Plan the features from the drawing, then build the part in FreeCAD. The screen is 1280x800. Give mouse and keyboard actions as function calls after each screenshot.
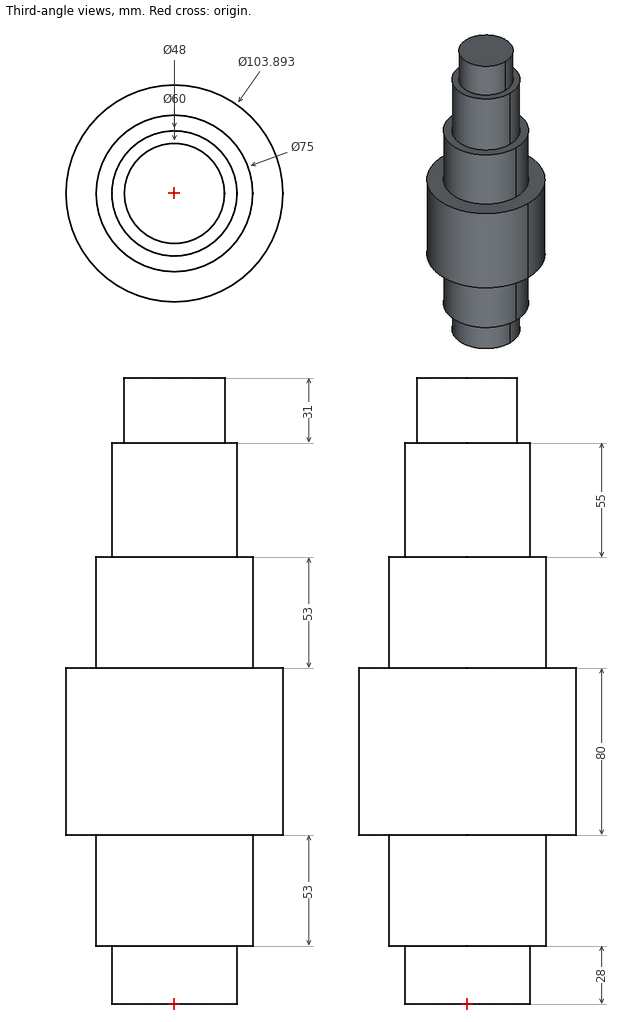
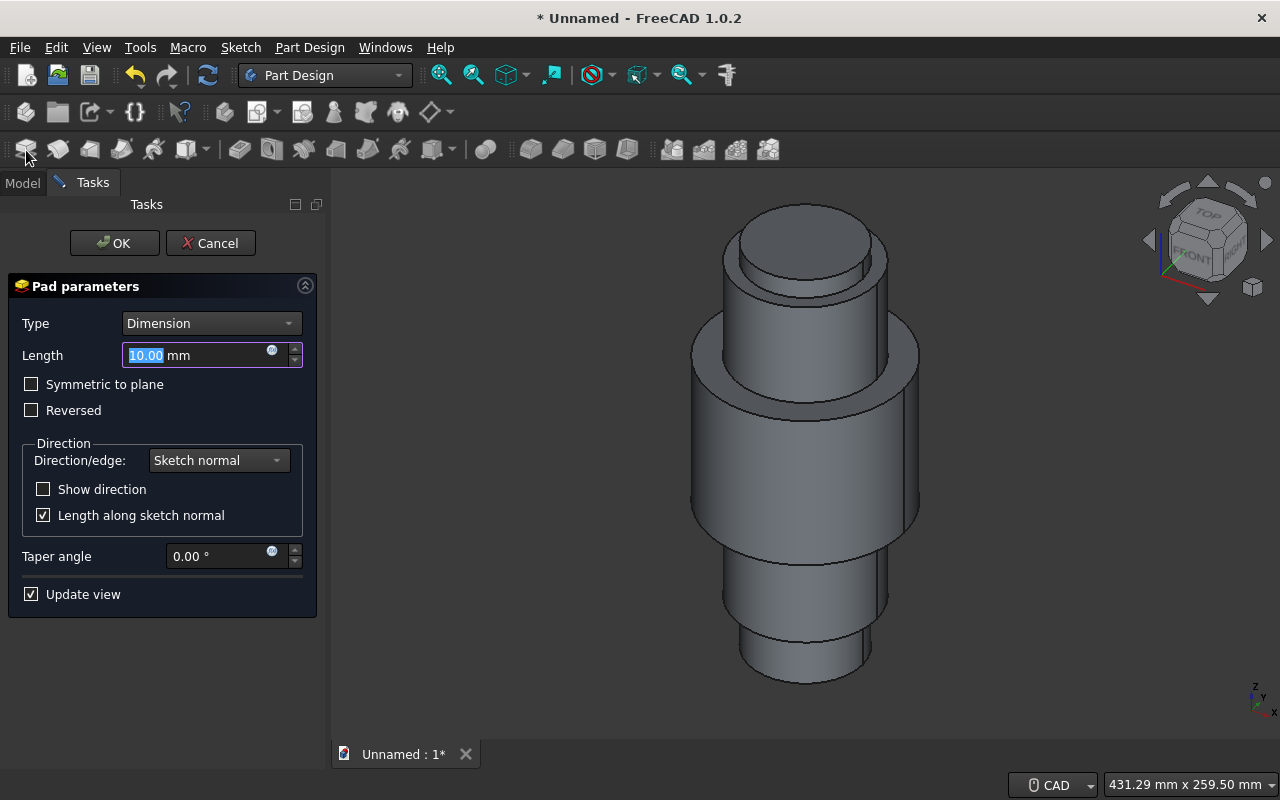
text(55)
key(Tab)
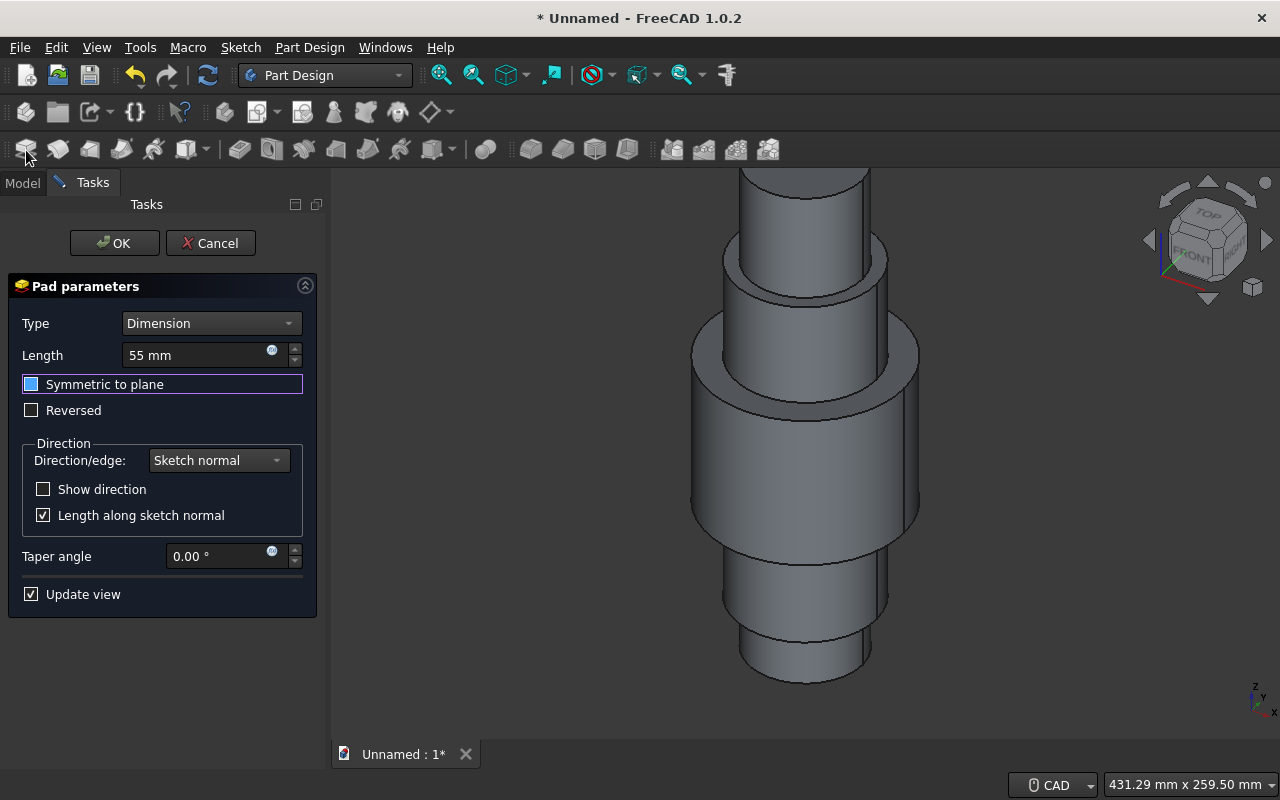
click(115, 243)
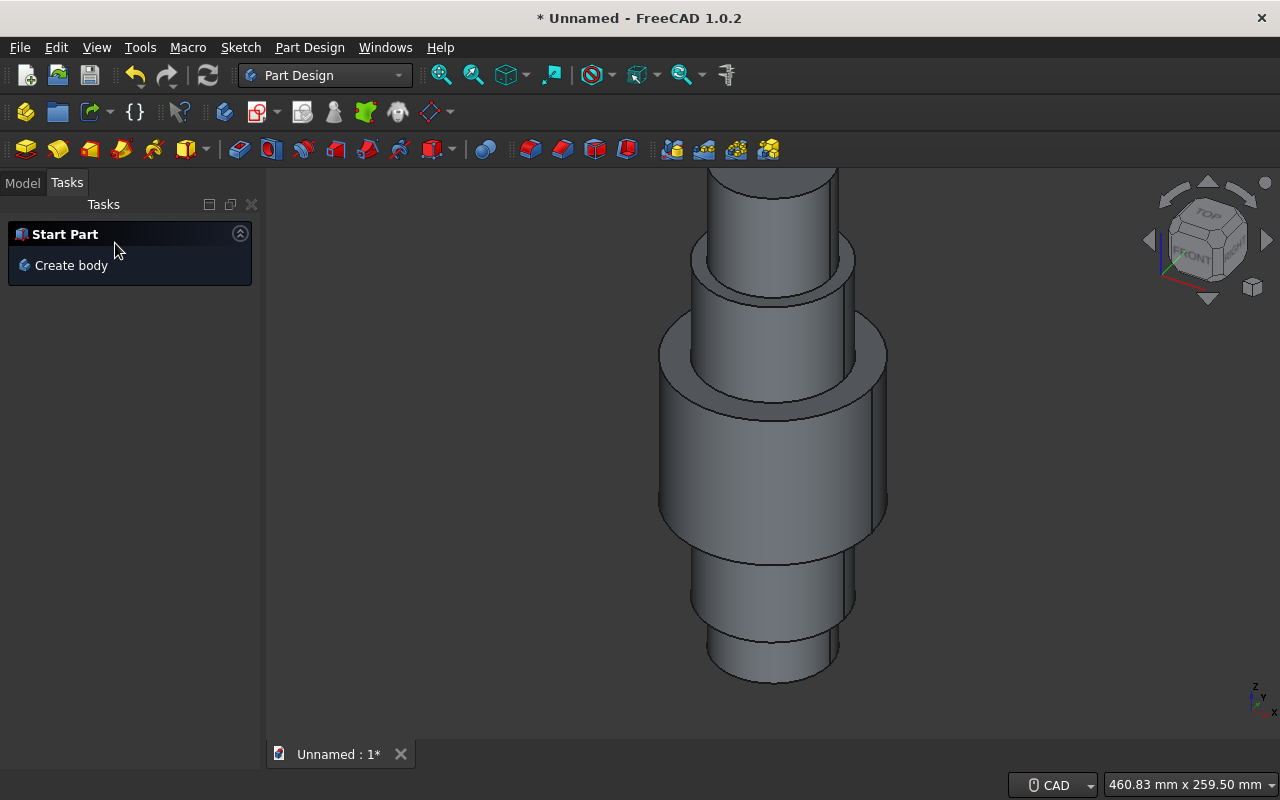
click(442, 76)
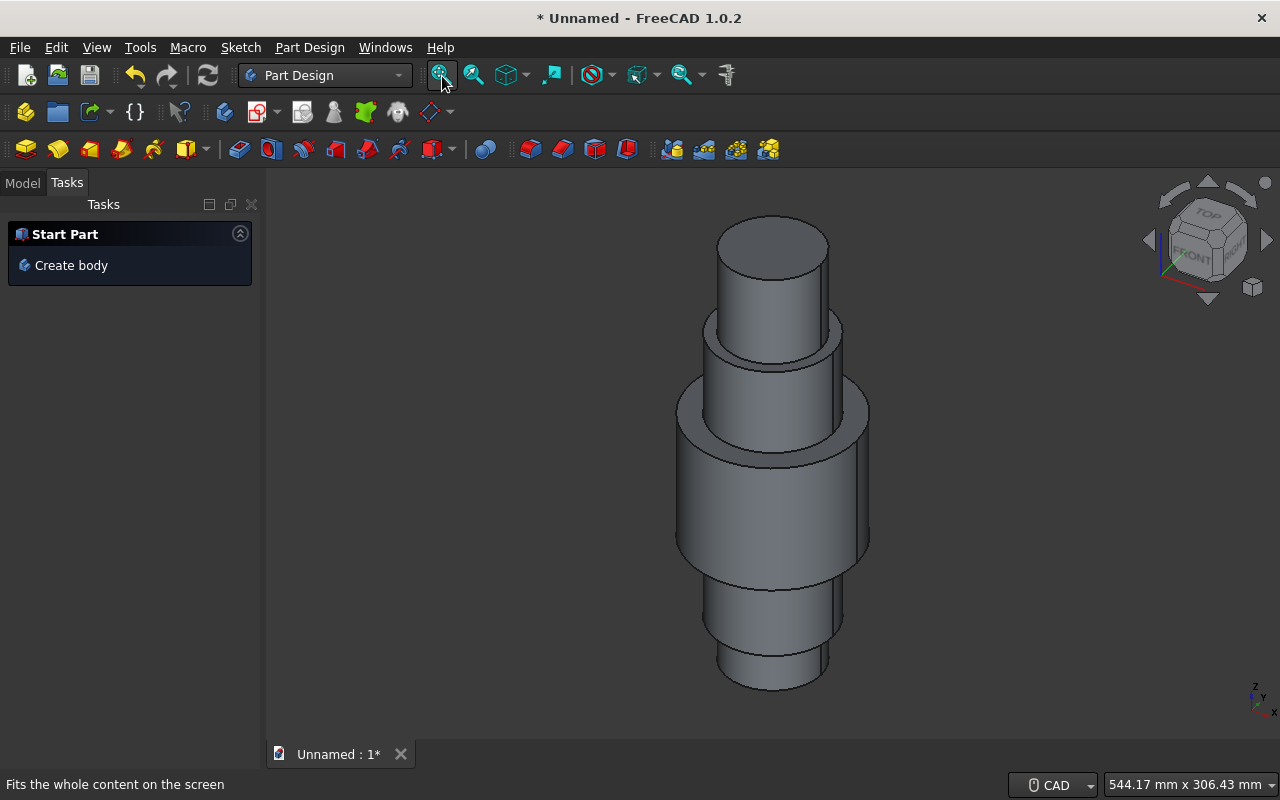
click(773, 247)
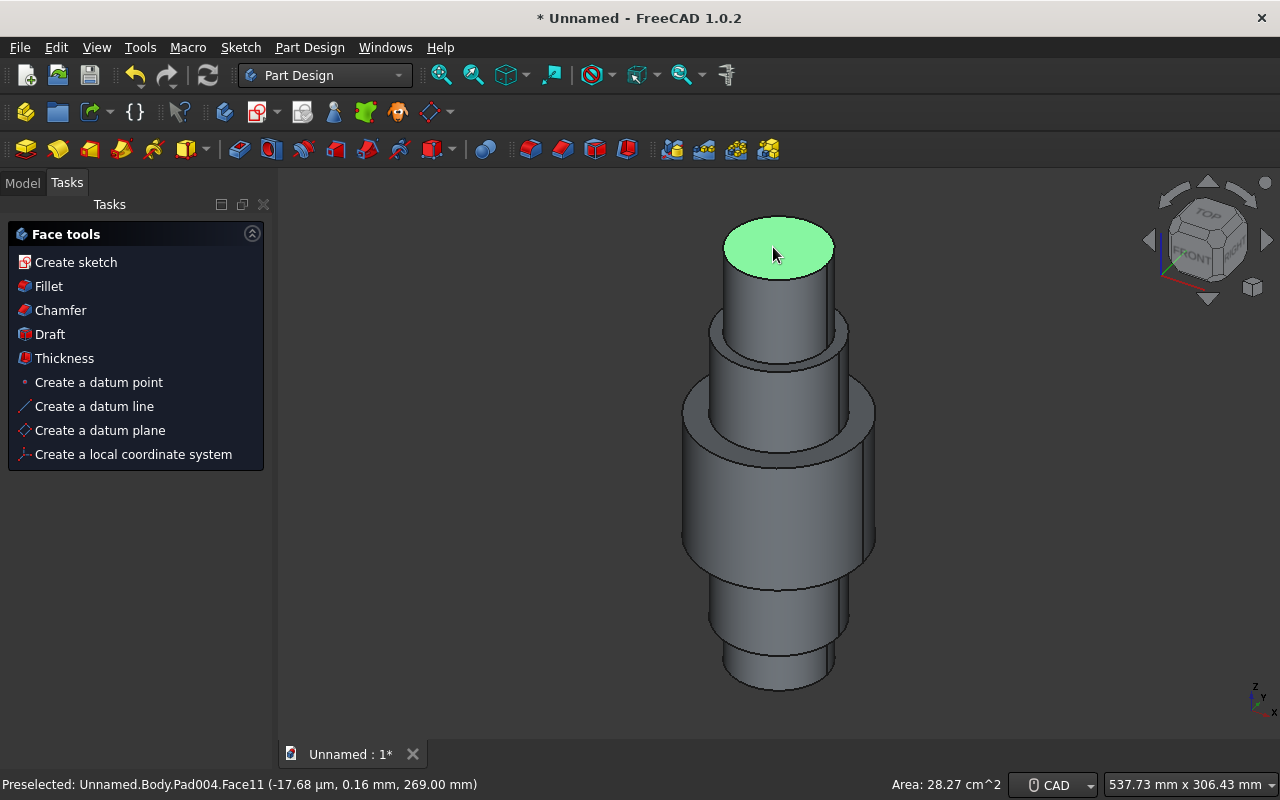
click(258, 112)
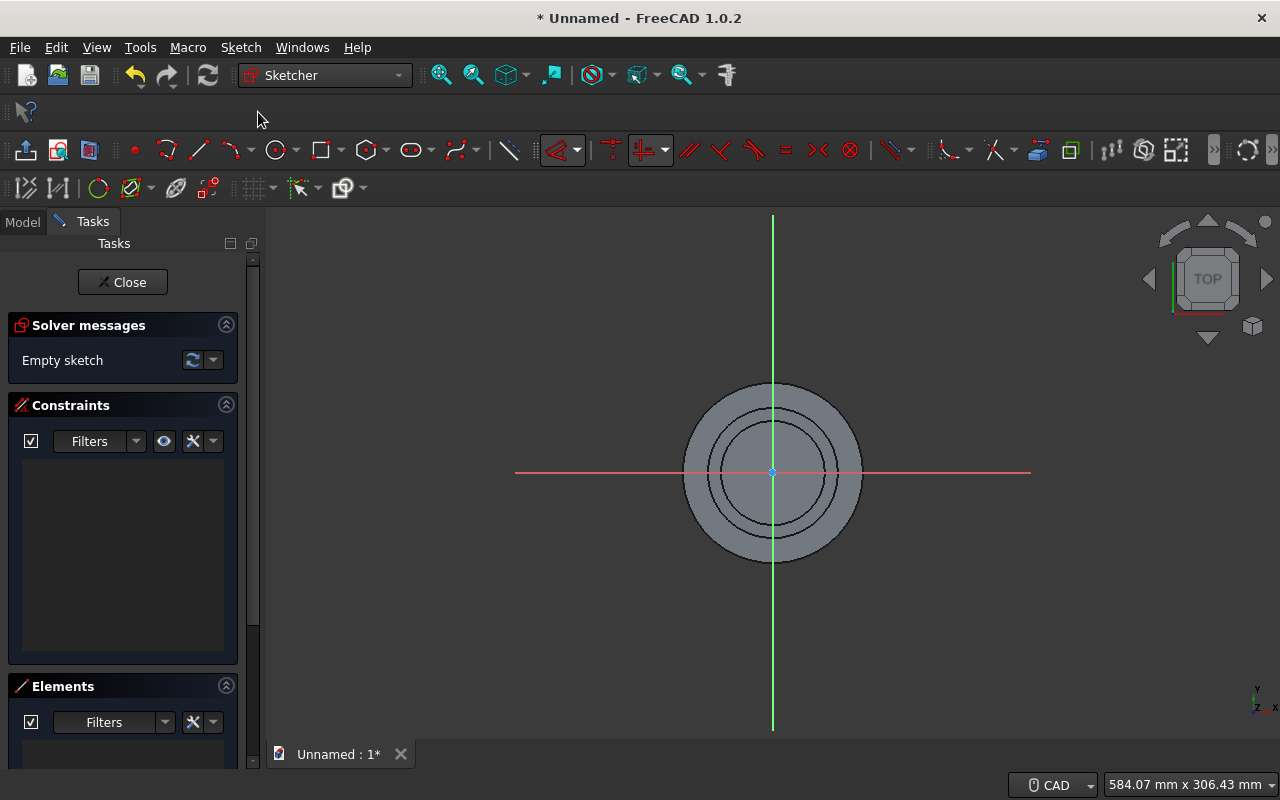
scroll(795, 473, up, 7)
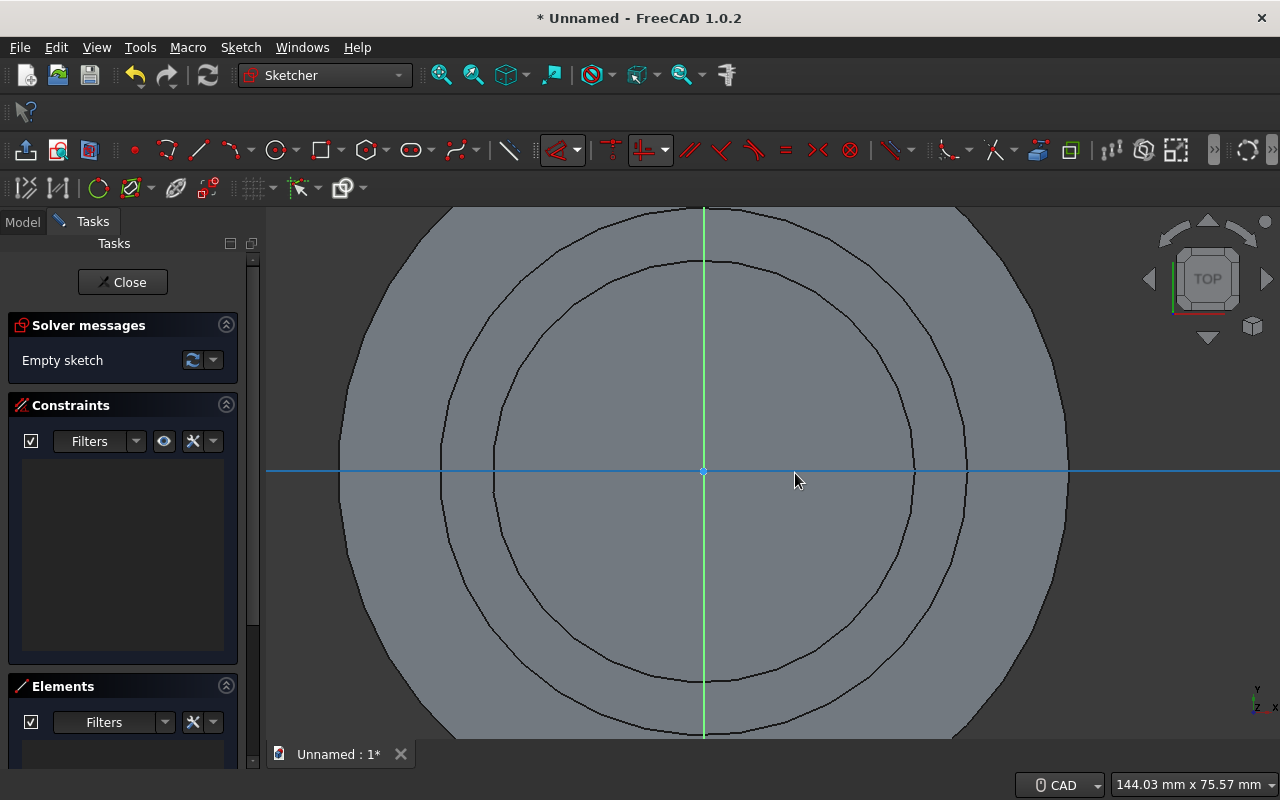
click(276, 150)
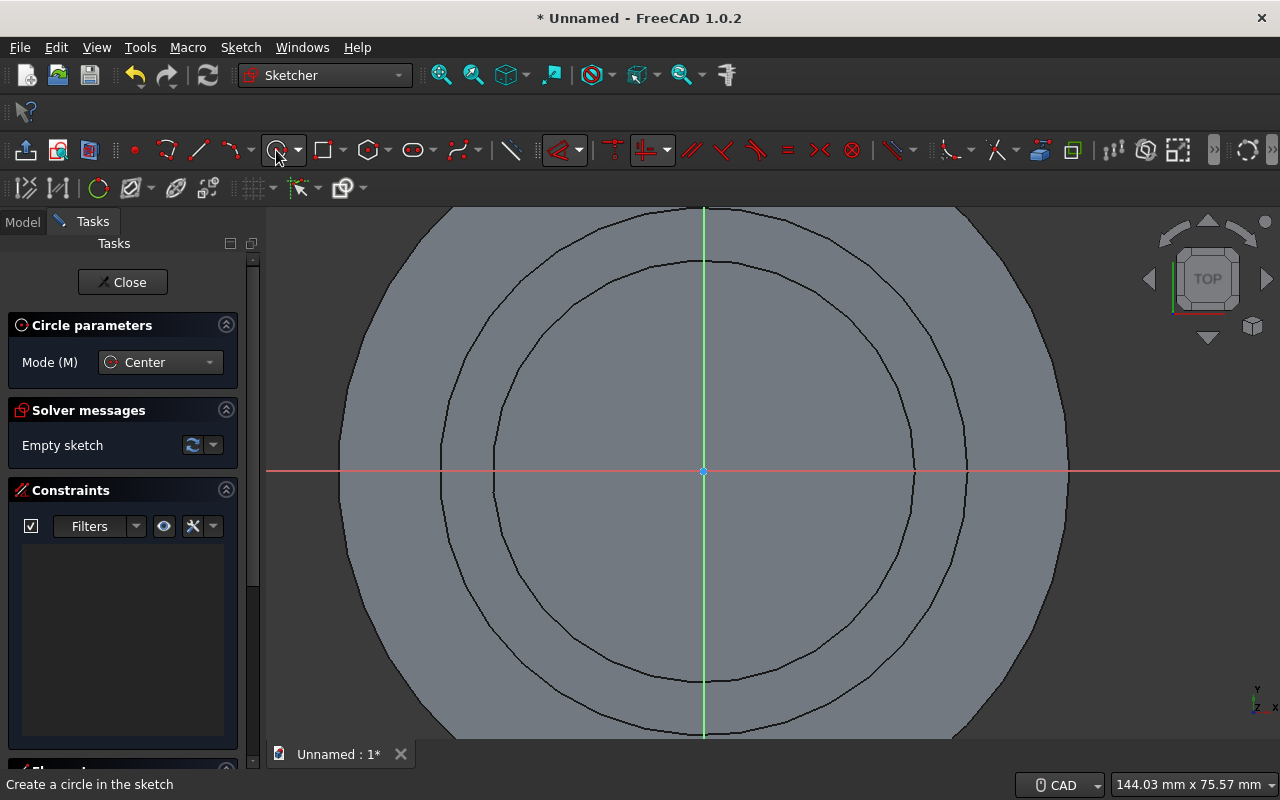
click(704, 471)
move(823, 352)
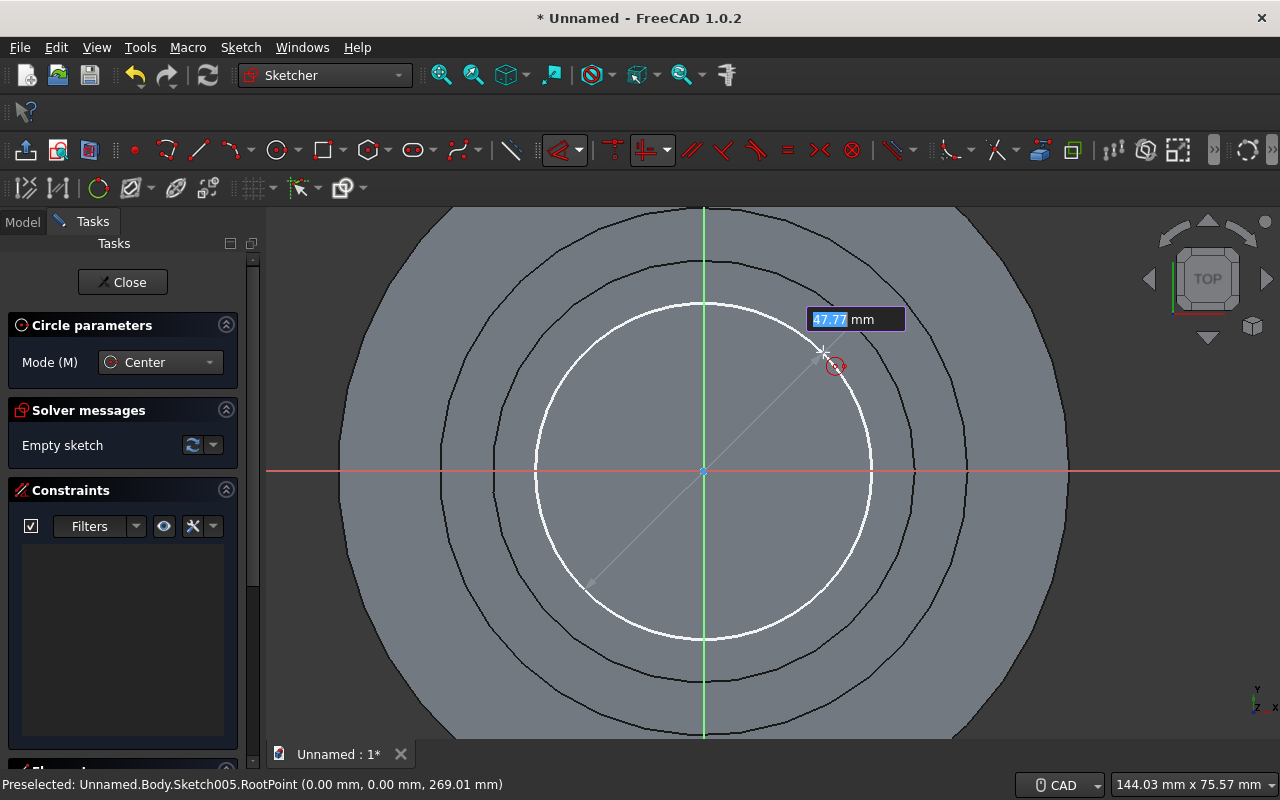
text(48)
key(Return)
key(Escape)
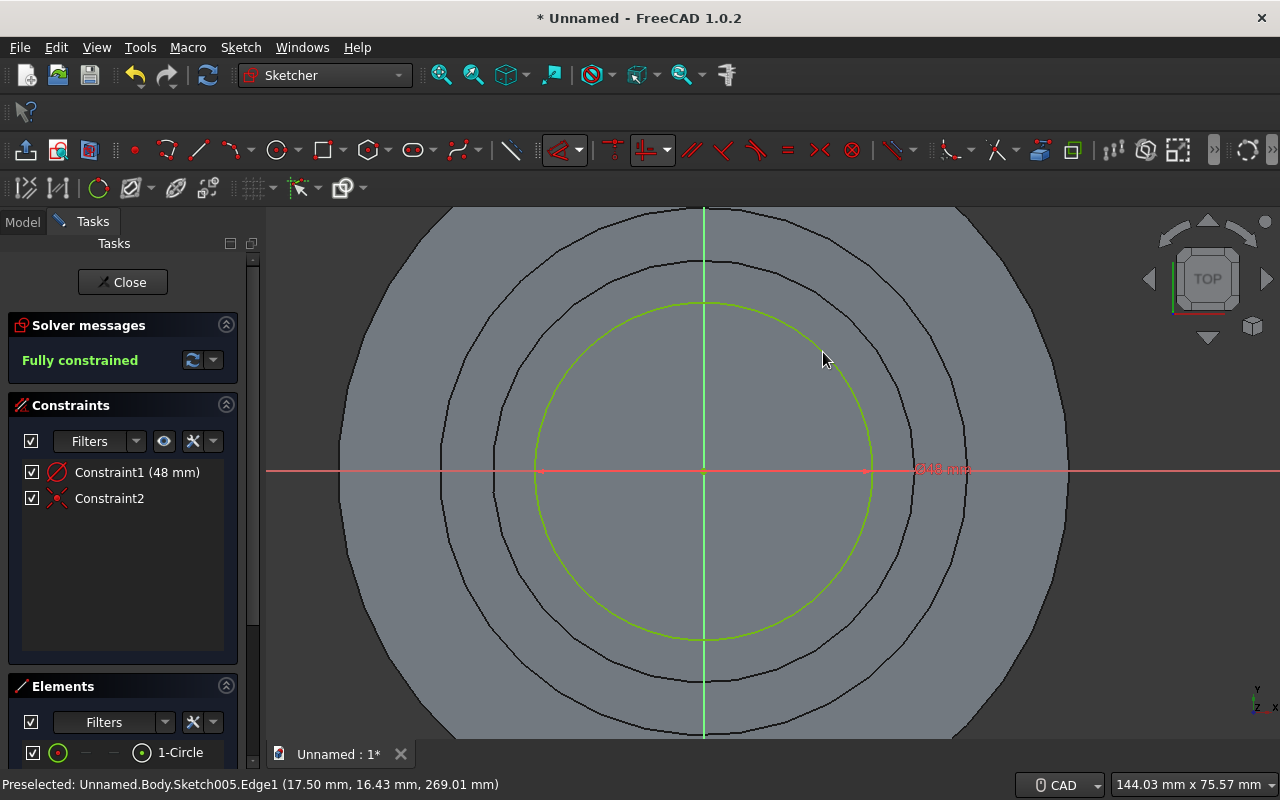
click(123, 282)